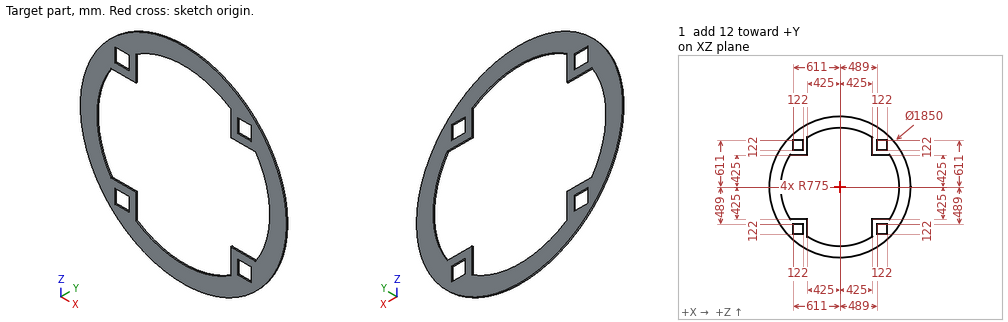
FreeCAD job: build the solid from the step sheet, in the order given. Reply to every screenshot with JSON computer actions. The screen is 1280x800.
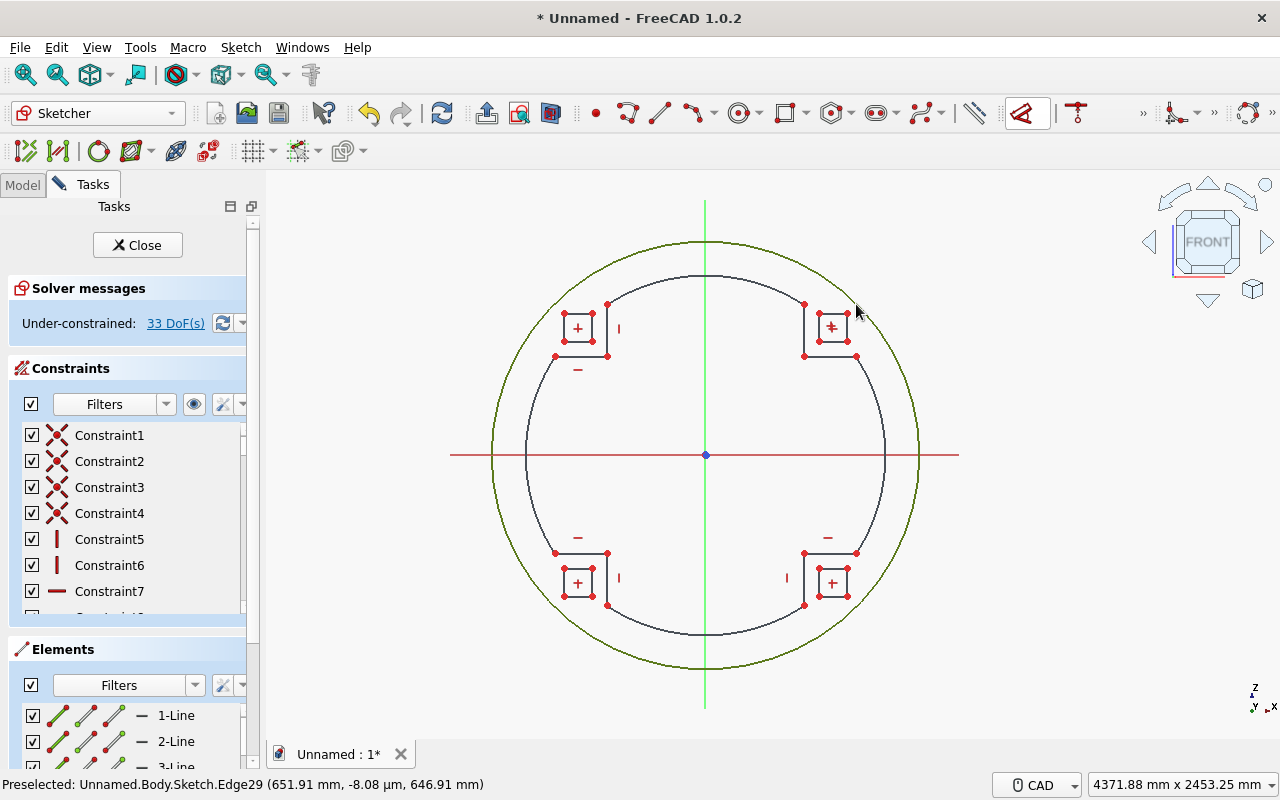
{"action": "left_click", "coordinate": [531, 414]}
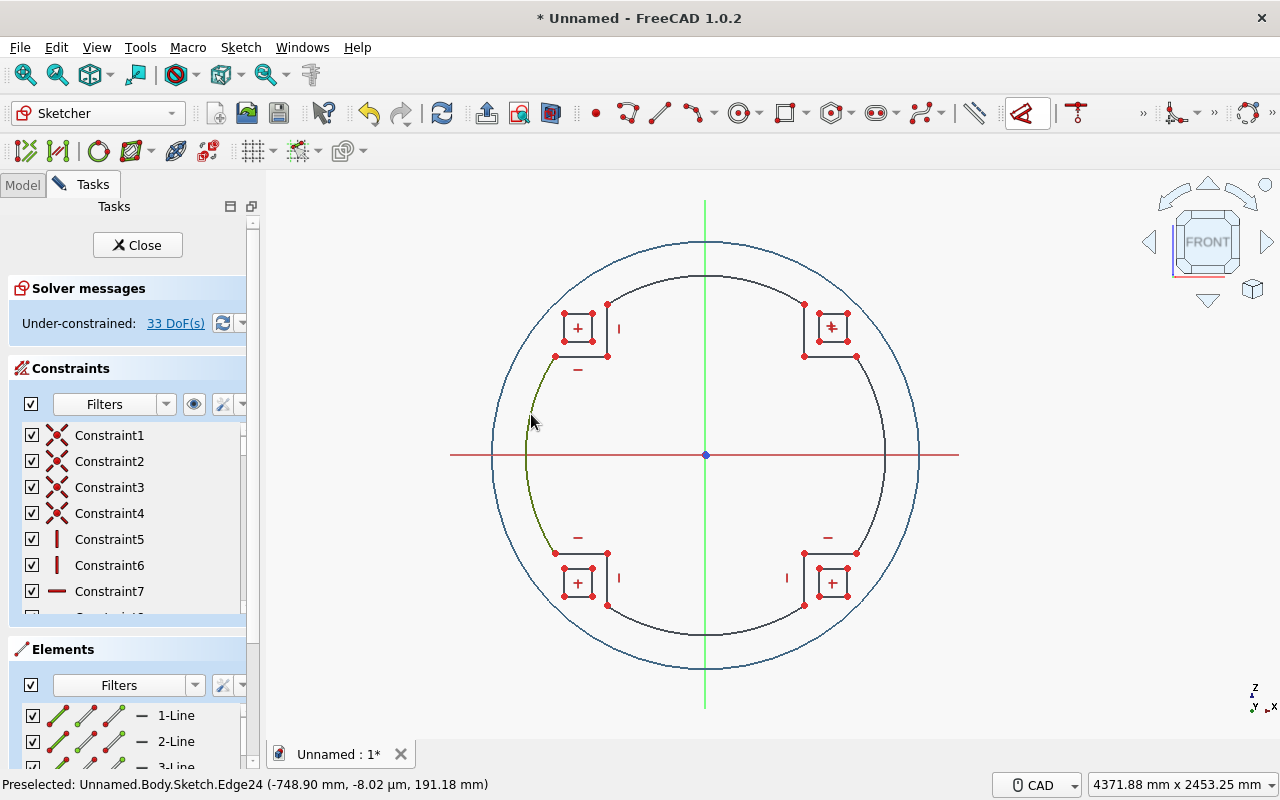
{"action": "left_click", "coordinate": [1076, 114]}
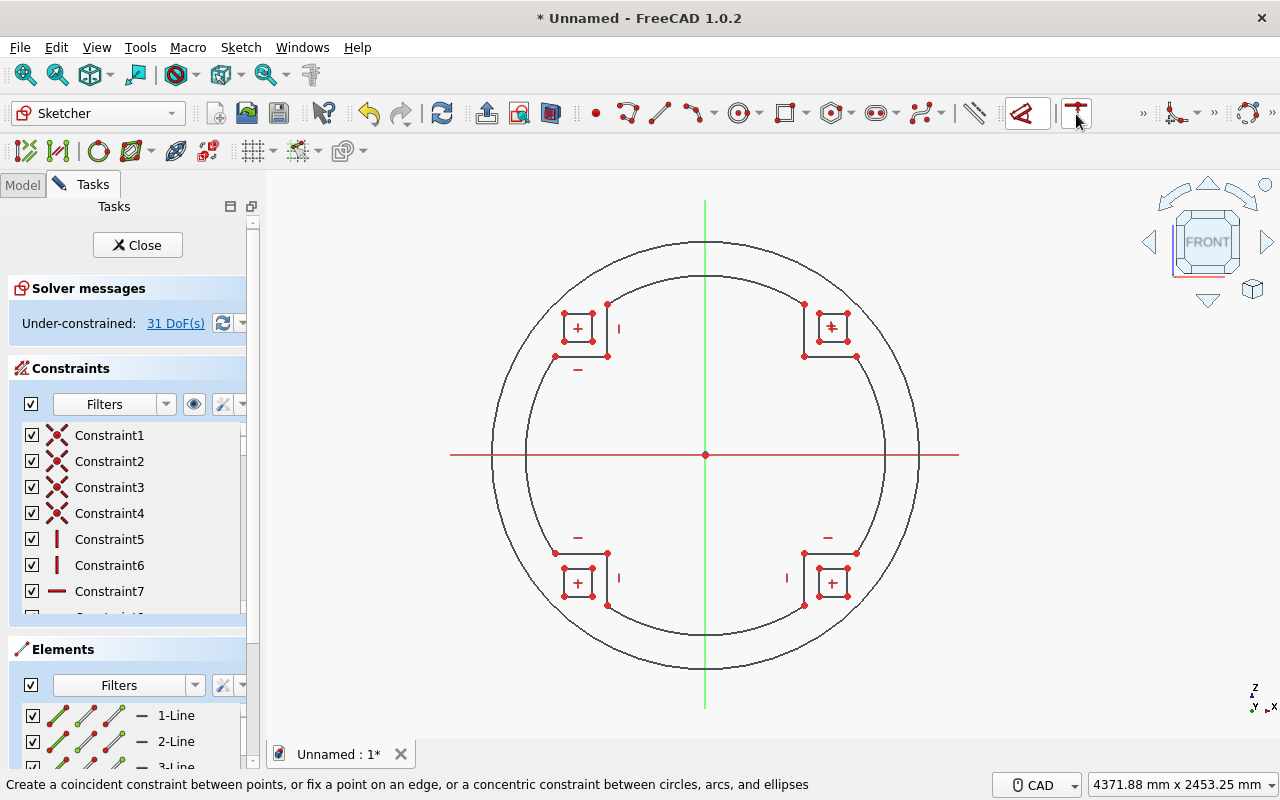
{"action": "left_click_drag", "start_coordinate": [695, 444], "coordinate": [716, 465]}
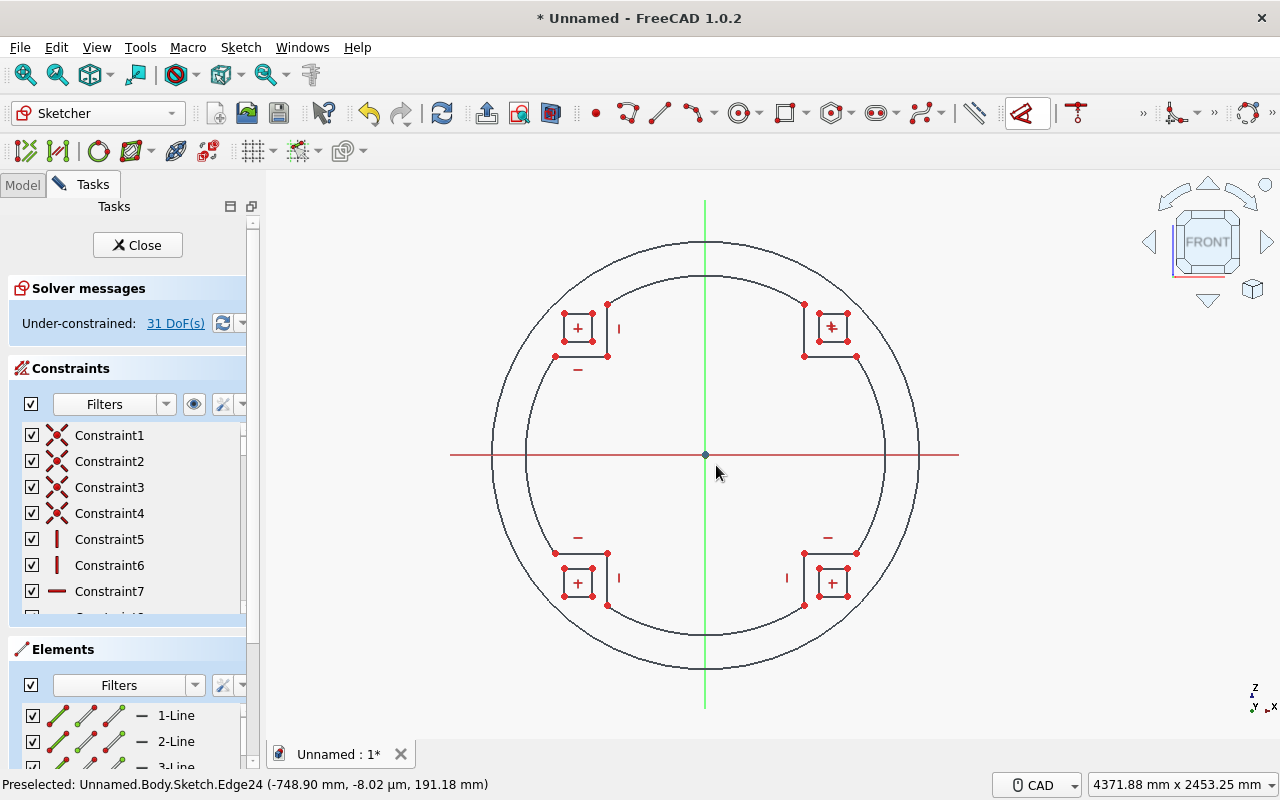
{"action": "left_click", "coordinate": [1076, 114]}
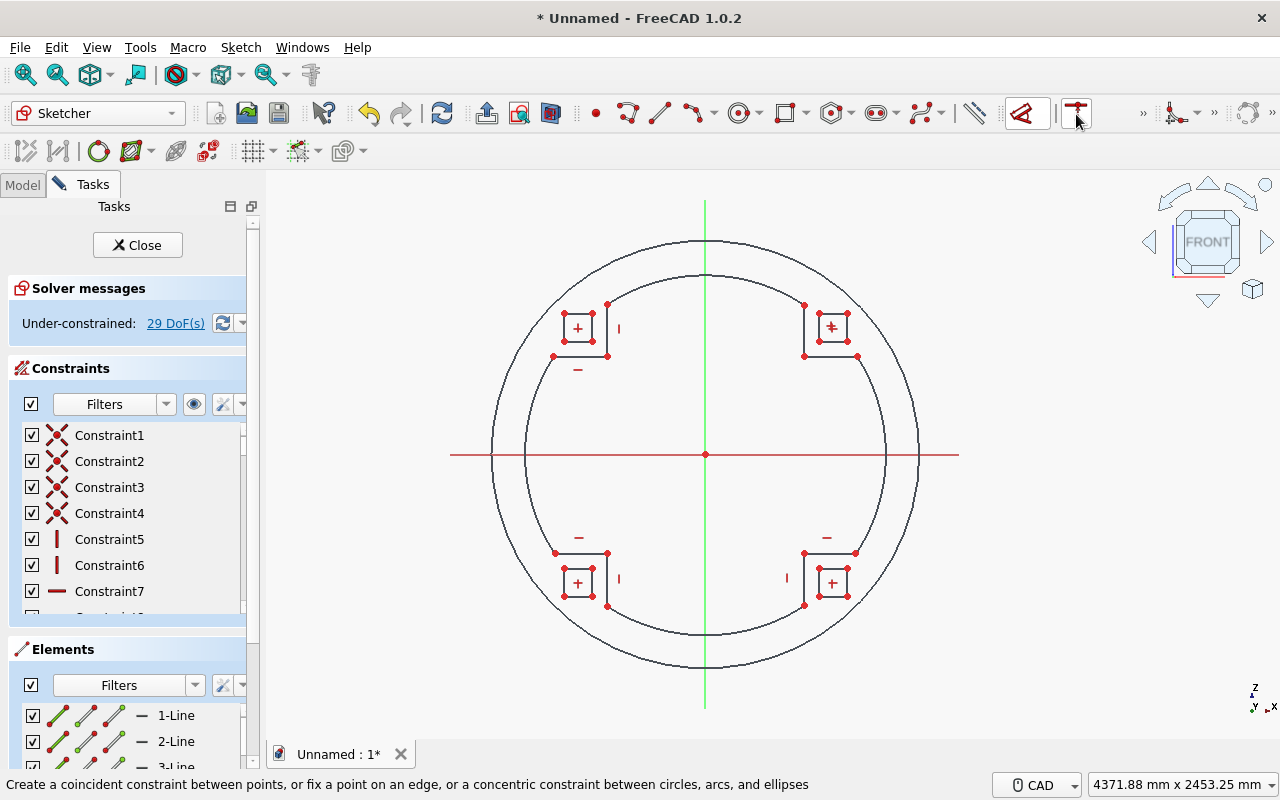
{"action": "left_click", "coordinate": [664, 631]}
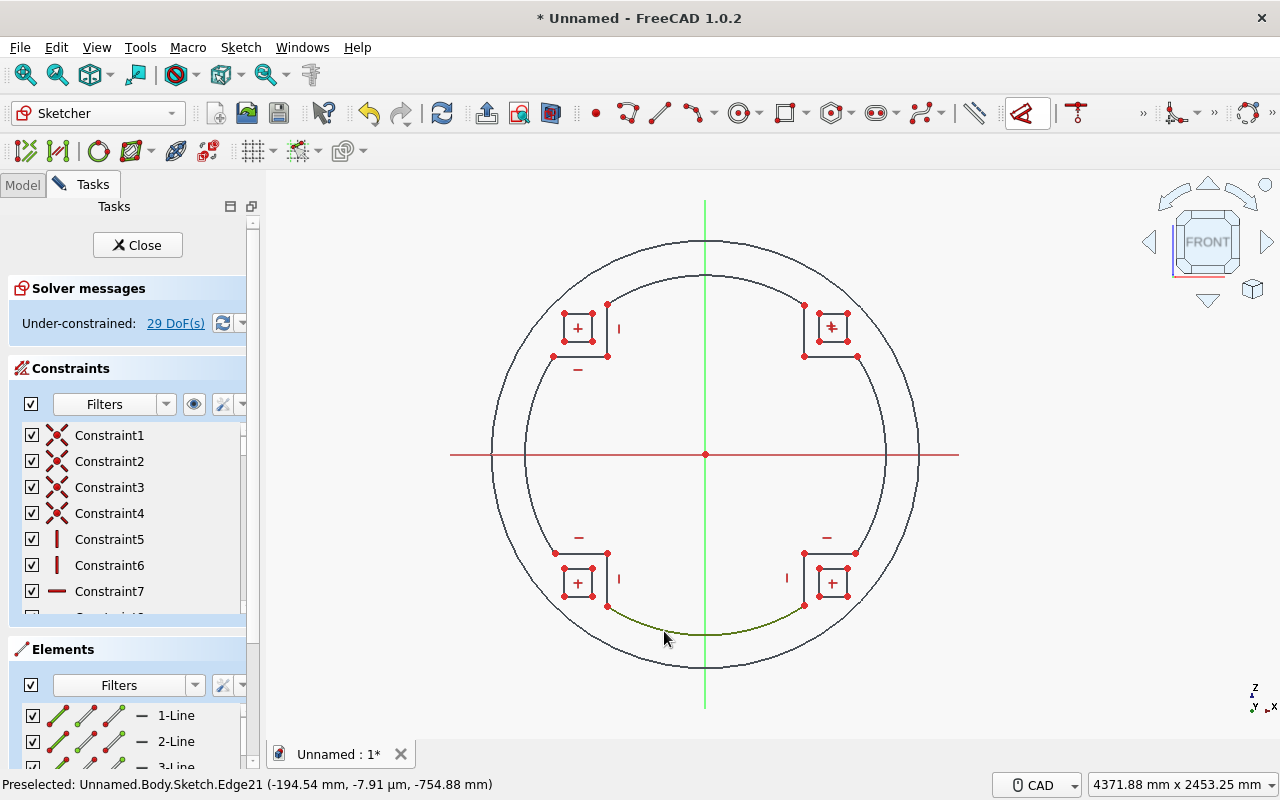
{"action": "left_click", "coordinate": [881, 497]}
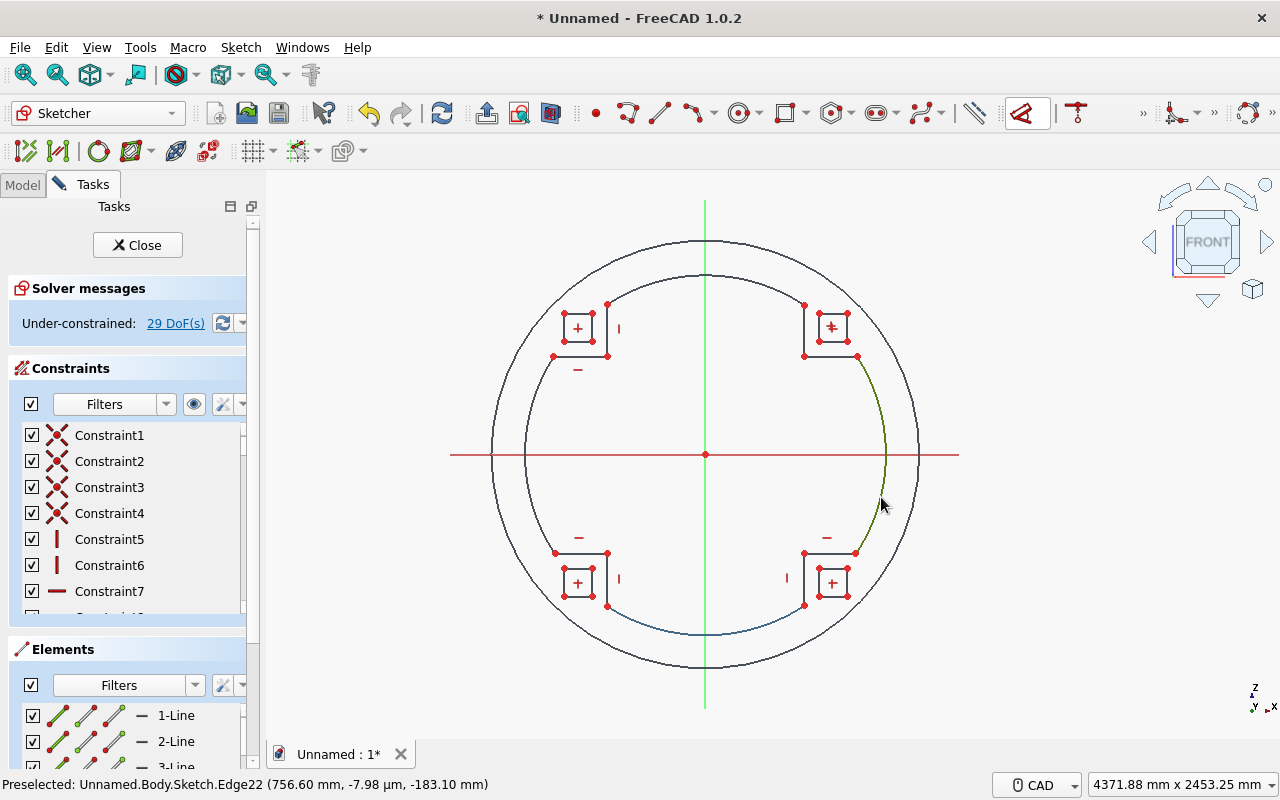
{"action": "left_click", "coordinate": [747, 280]}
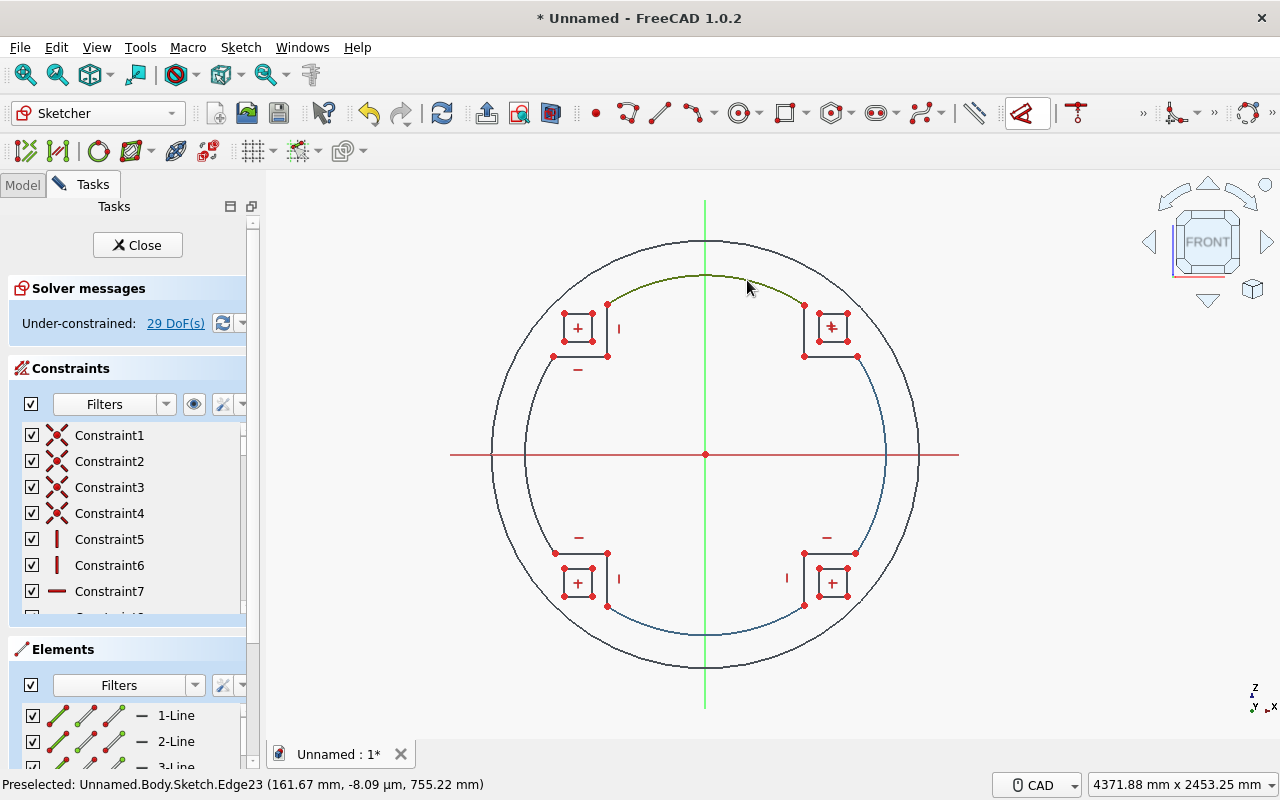
{"action": "left_click", "coordinate": [530, 414]}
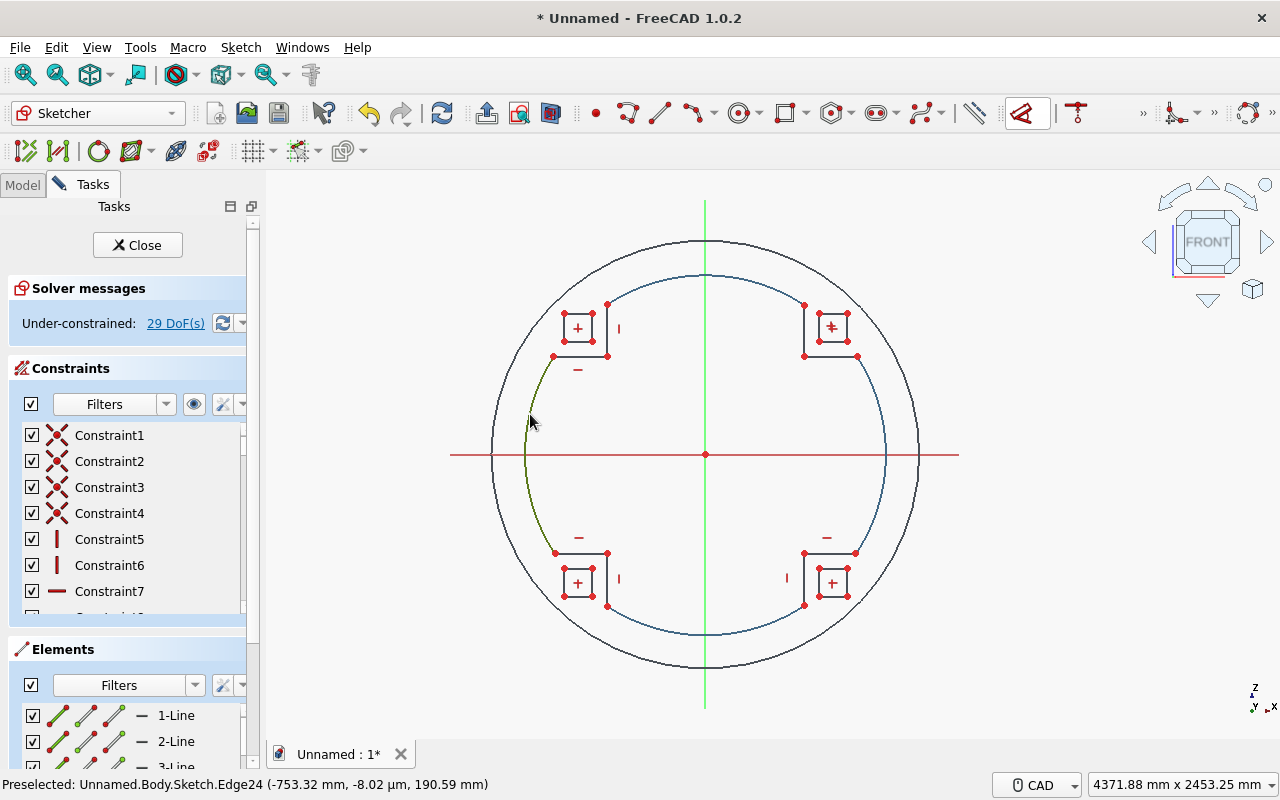
{"action": "key", "text": "e"}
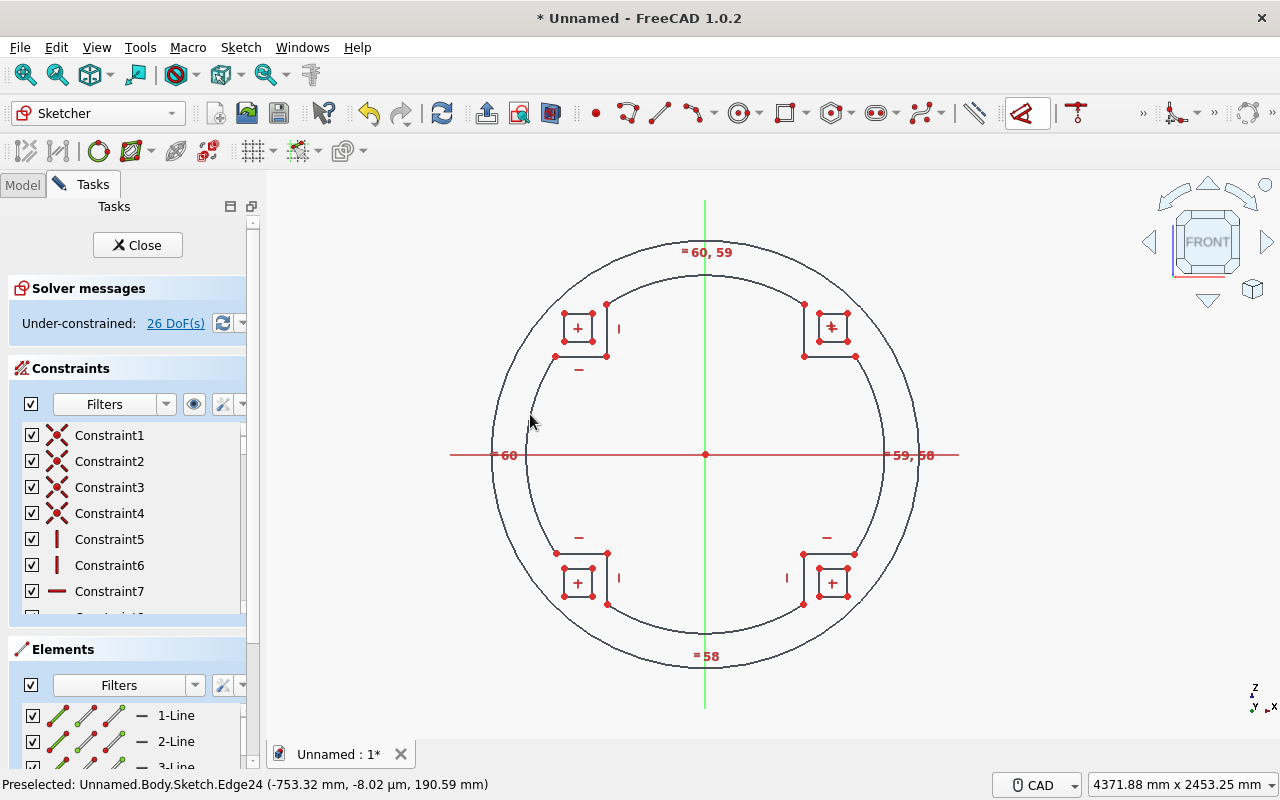
{"action": "left_click", "coordinate": [664, 629]}